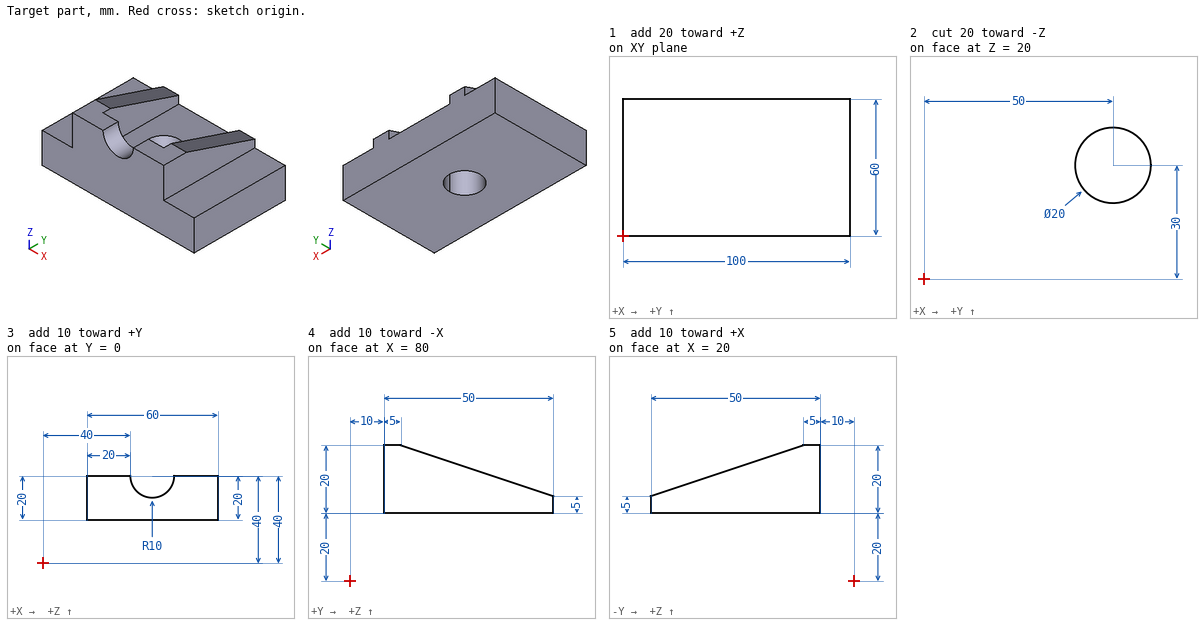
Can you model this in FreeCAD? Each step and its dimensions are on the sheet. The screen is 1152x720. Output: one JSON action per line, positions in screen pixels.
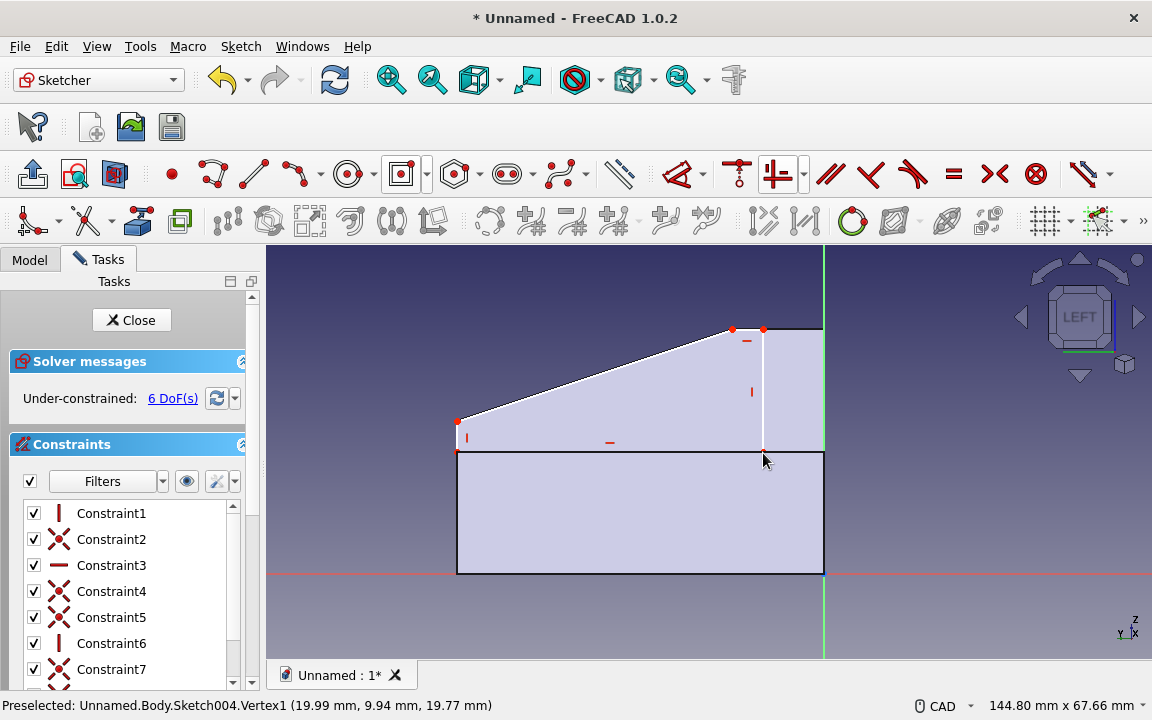
{"action": "left_click", "coordinate": [676, 174]}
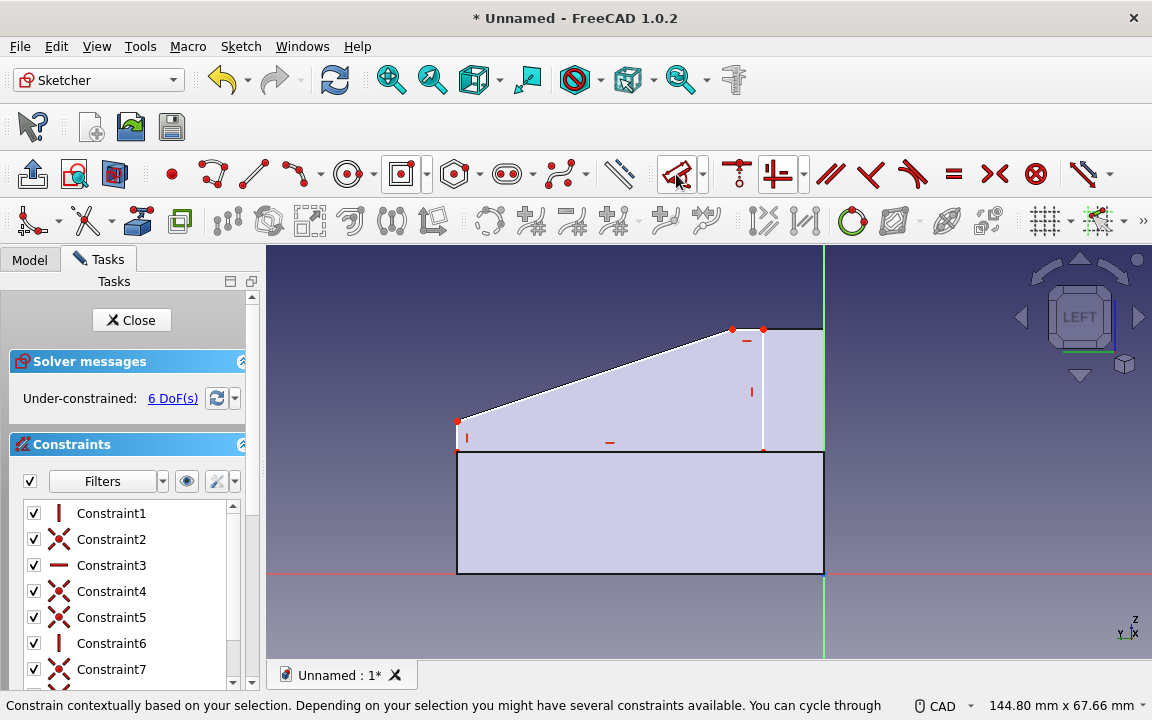
{"action": "scroll", "coordinate": [754, 330], "scroll_direction": "up", "scroll_amount": 2}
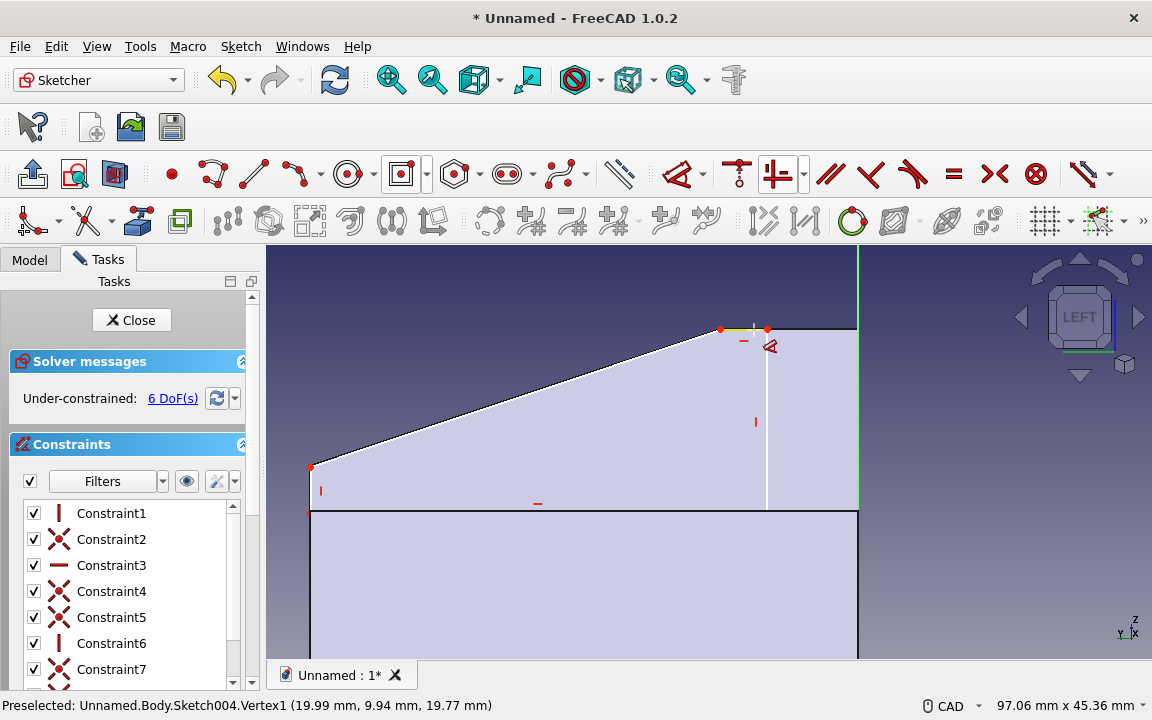
{"action": "left_click", "coordinate": [753, 330]}
{"action": "left_click", "coordinate": [744, 296]}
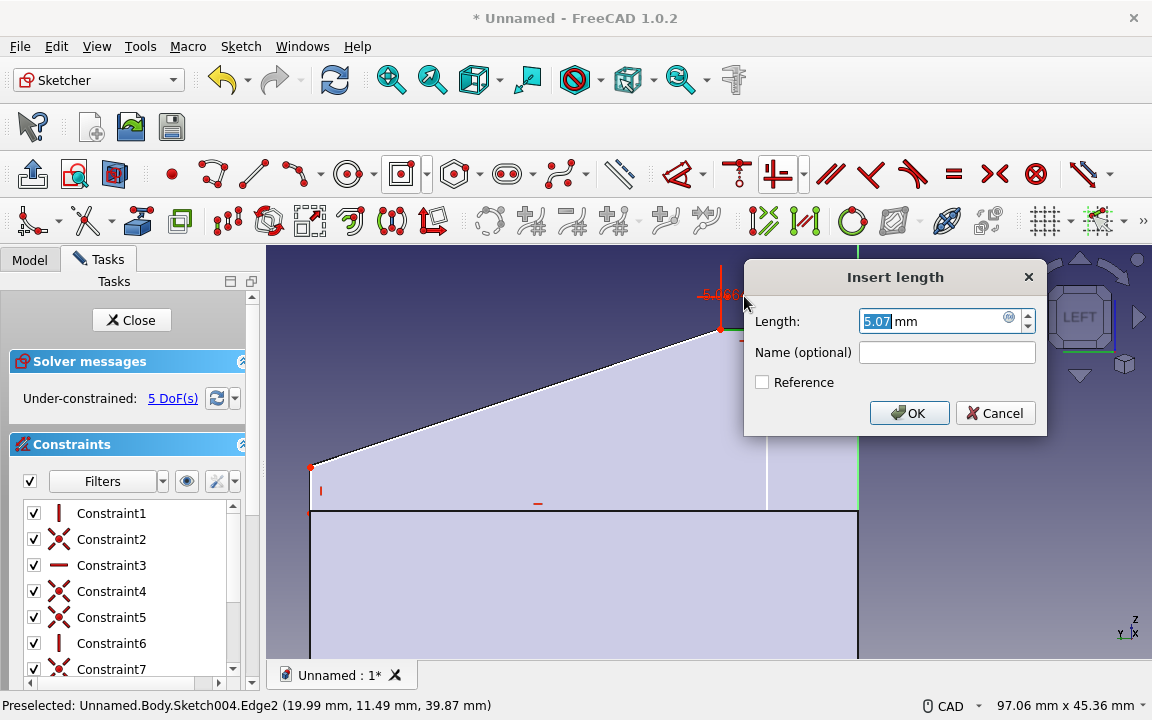
{"action": "type", "text": "5"}
{"action": "key", "text": "Return"}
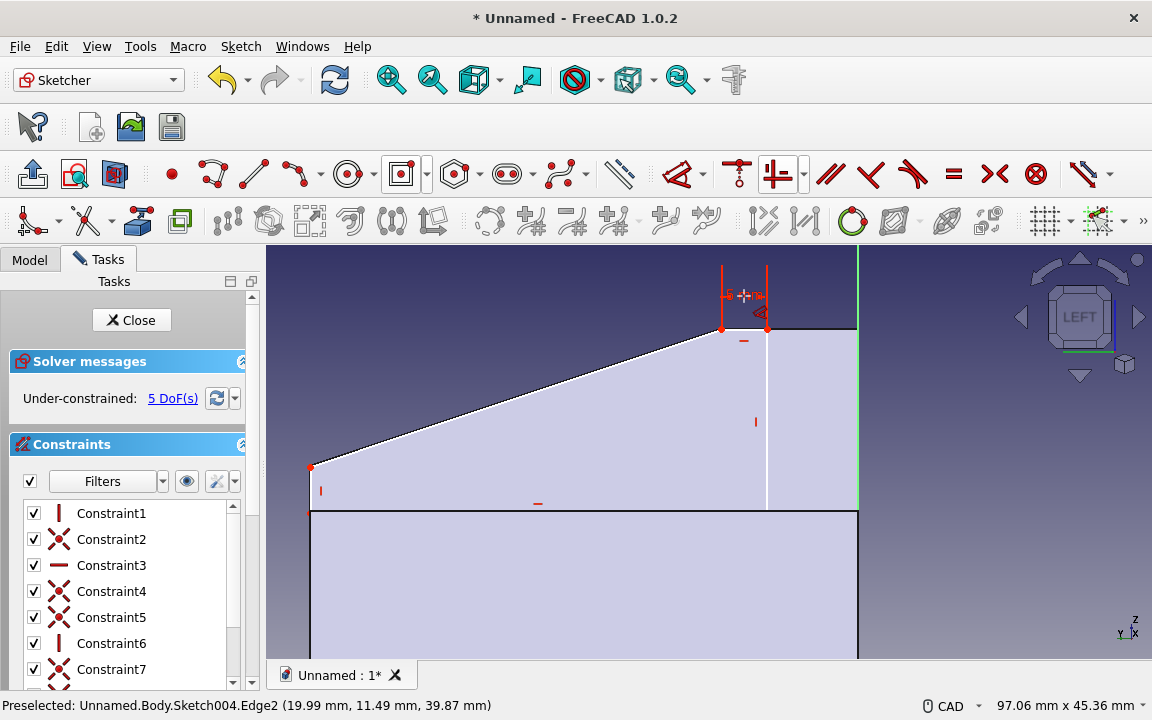
{"action": "left_click", "coordinate": [311, 481]}
{"action": "left_click", "coordinate": [345, 490]}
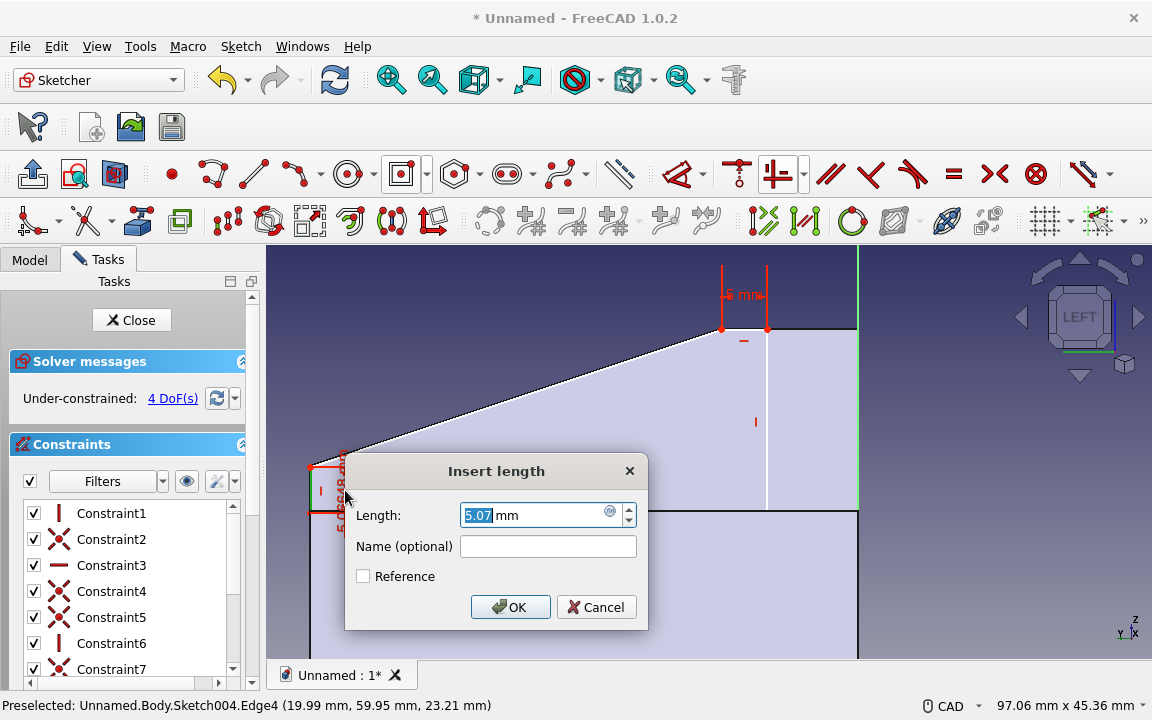
{"action": "type", "text": "5"}
{"action": "key", "text": "Return"}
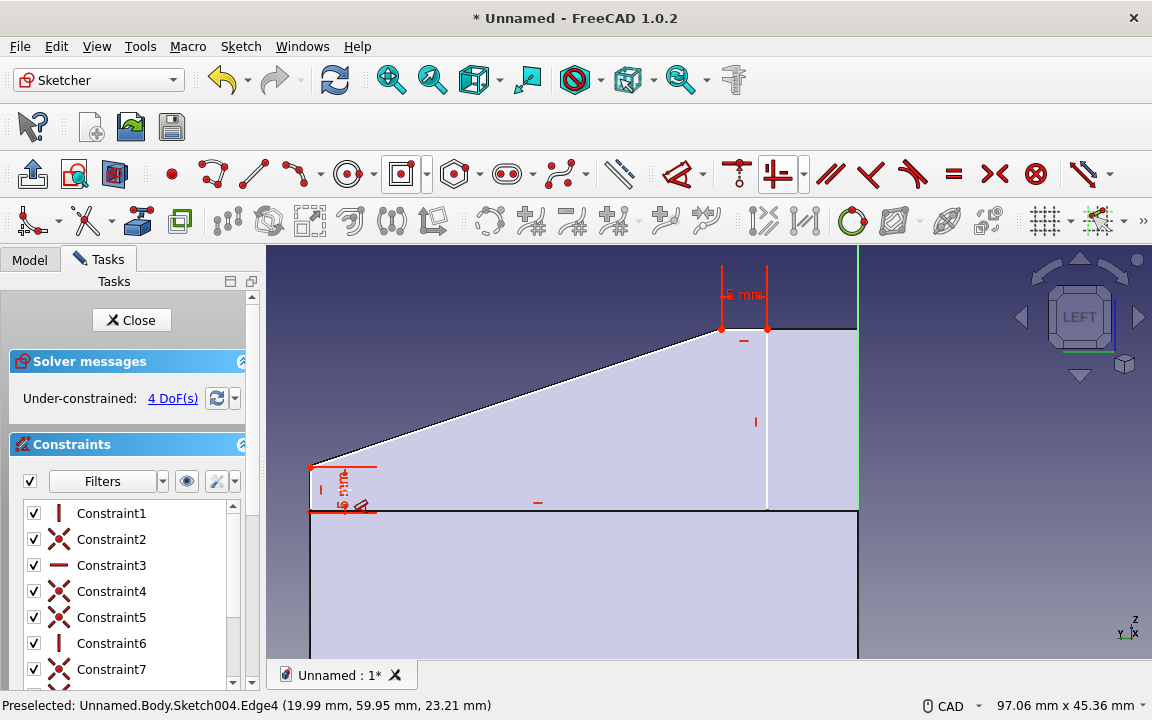
{"action": "left_click", "coordinate": [767, 458]}
{"action": "left_click", "coordinate": [801, 421]}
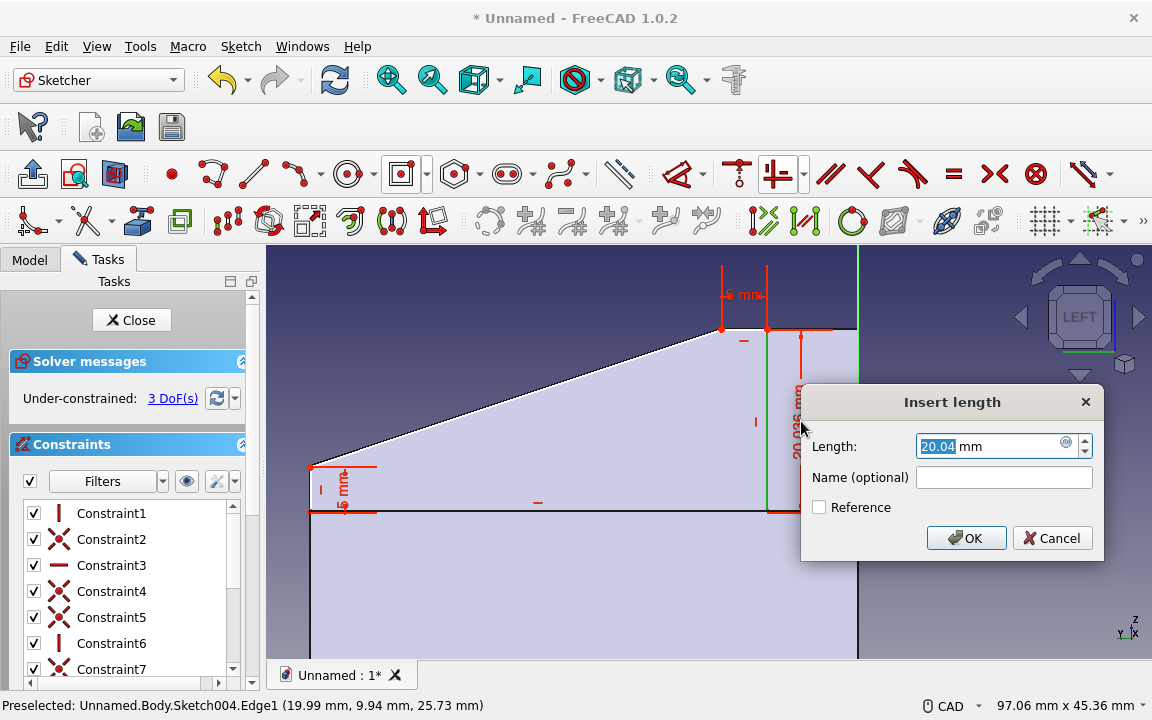
{"action": "type", "text": "20"}
{"action": "key", "text": "Return"}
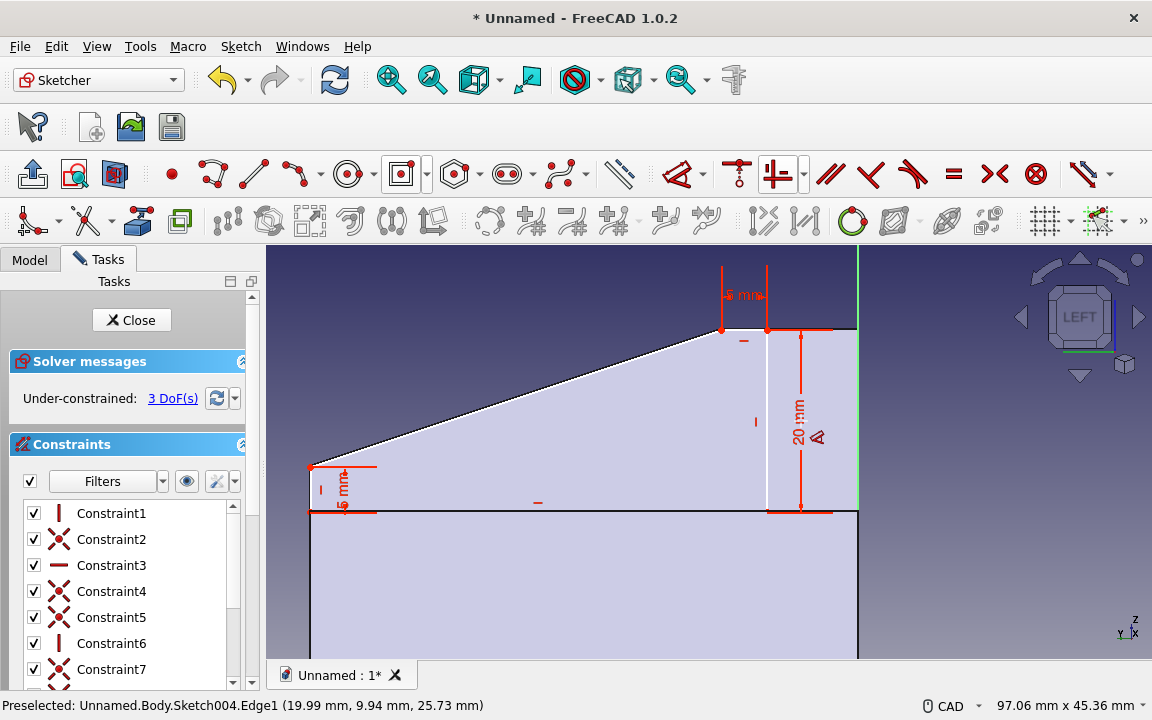
{"action": "left_click", "coordinate": [448, 513]}
{"action": "left_click", "coordinate": [539, 547]}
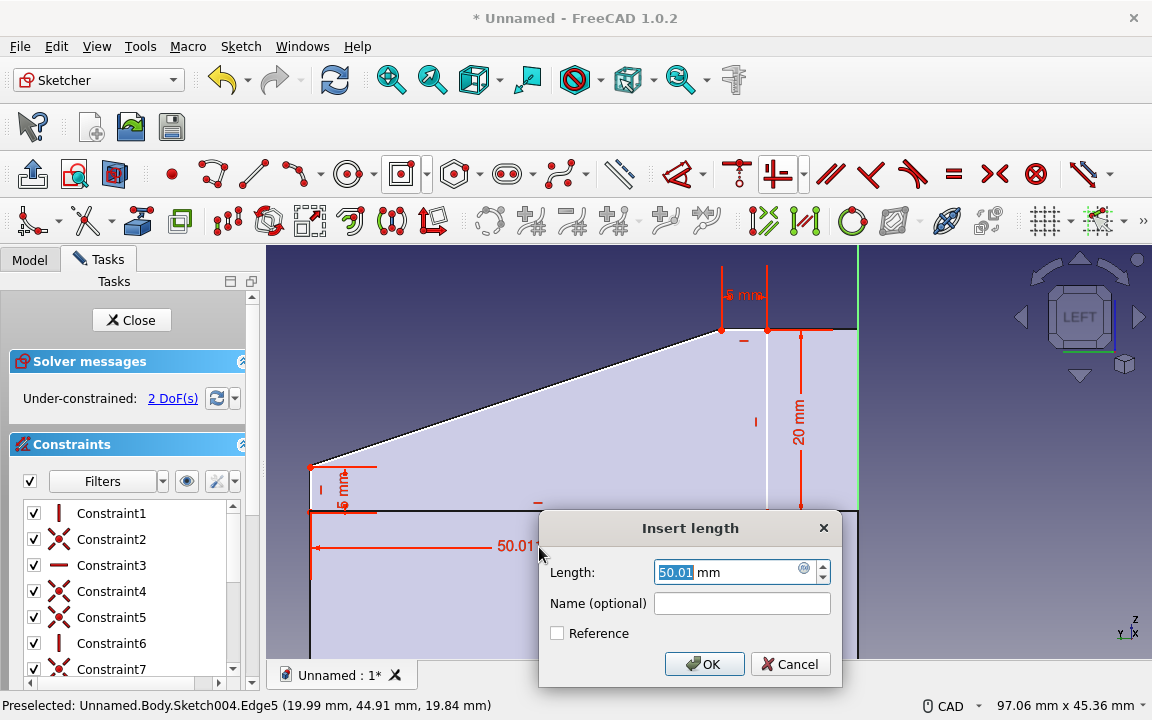
{"action": "type", "text": "50"}
{"action": "key", "text": "Return"}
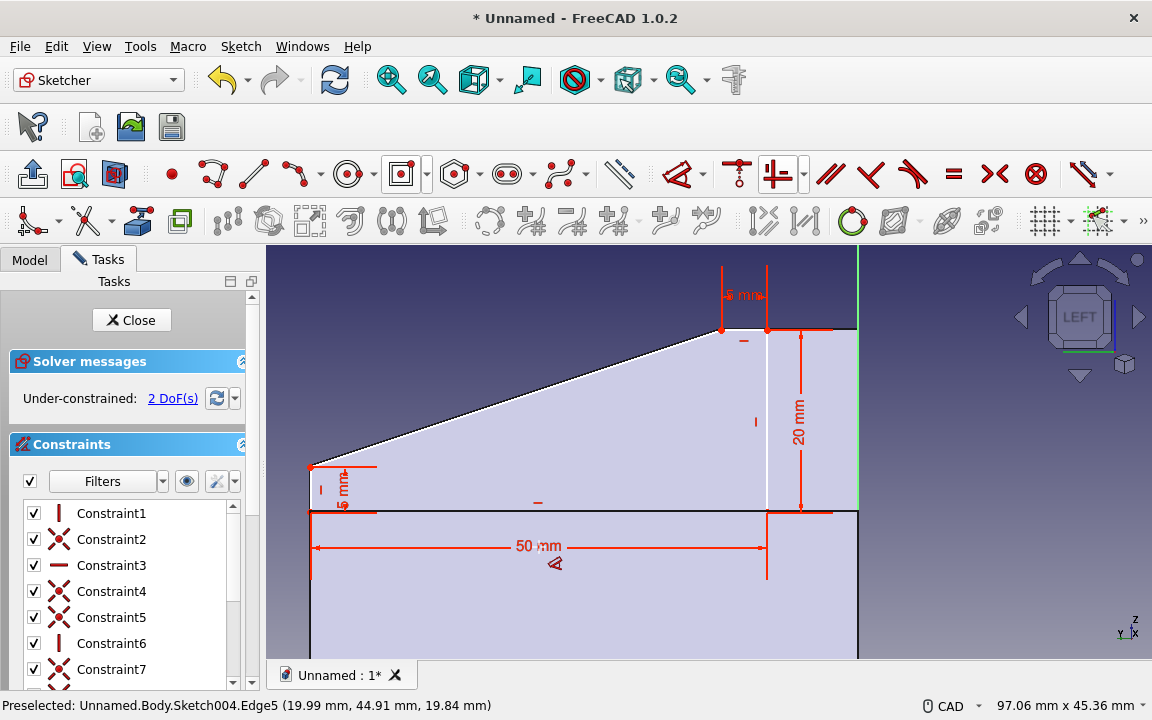
{"action": "left_click", "coordinate": [767, 513]}
{"action": "left_click", "coordinate": [813, 479]}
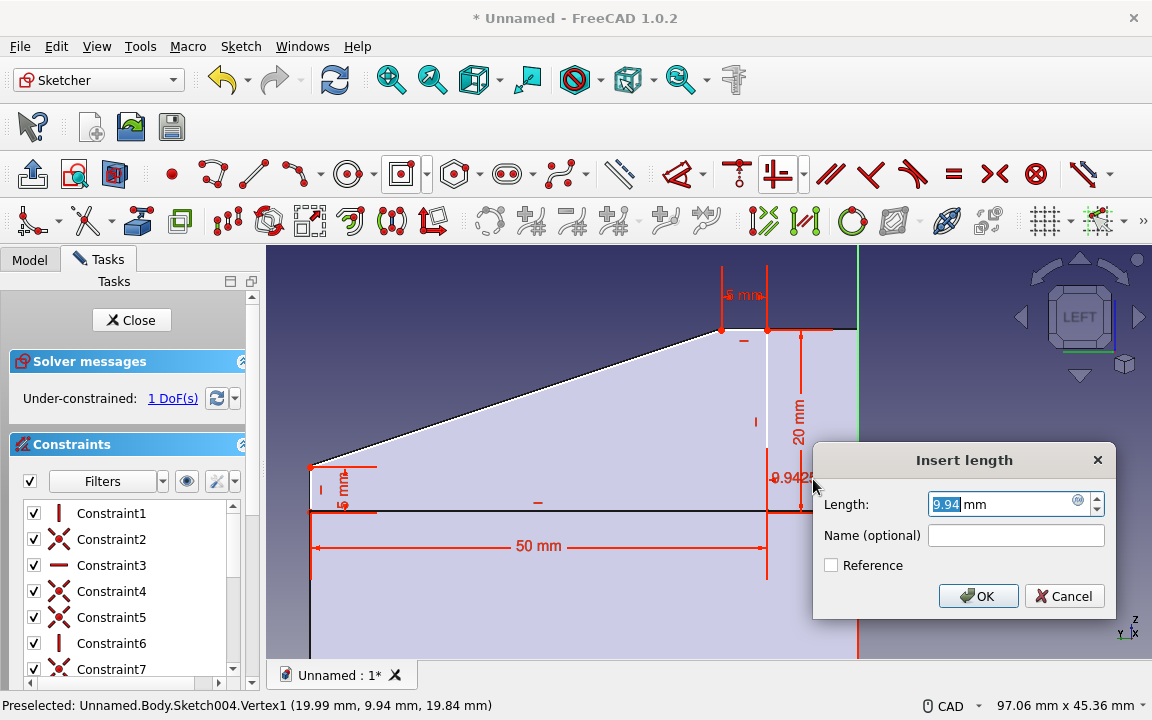
{"action": "type", "text": "10"}
{"action": "key", "text": "Return"}